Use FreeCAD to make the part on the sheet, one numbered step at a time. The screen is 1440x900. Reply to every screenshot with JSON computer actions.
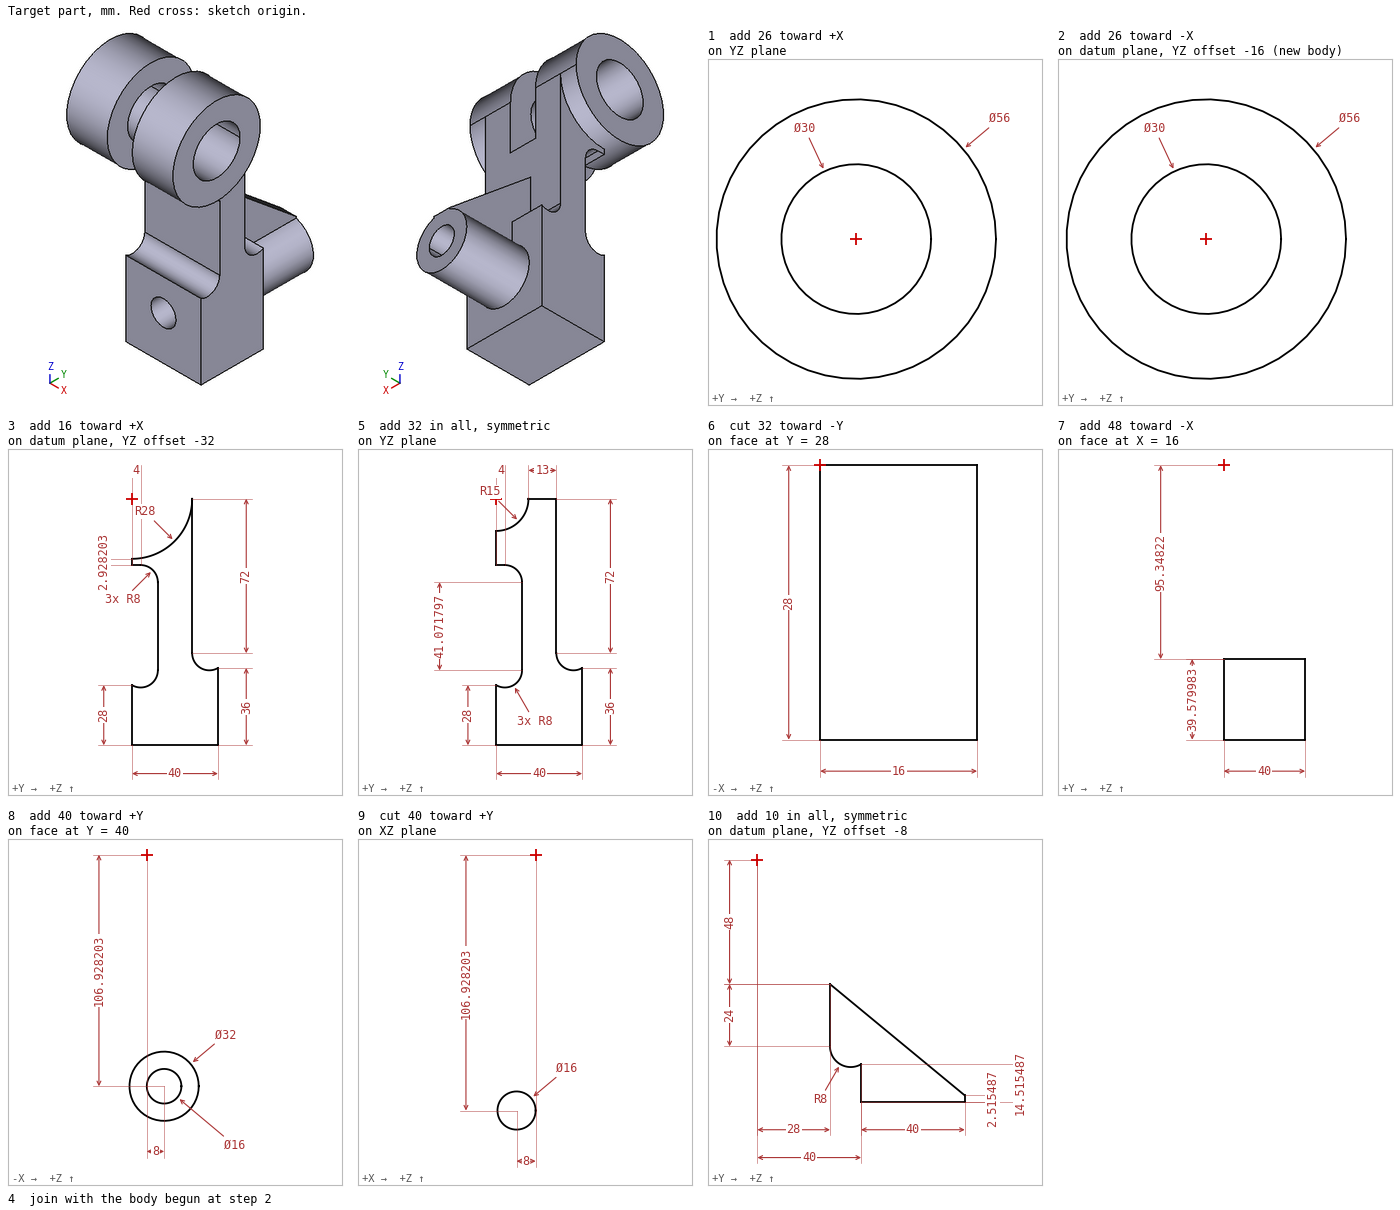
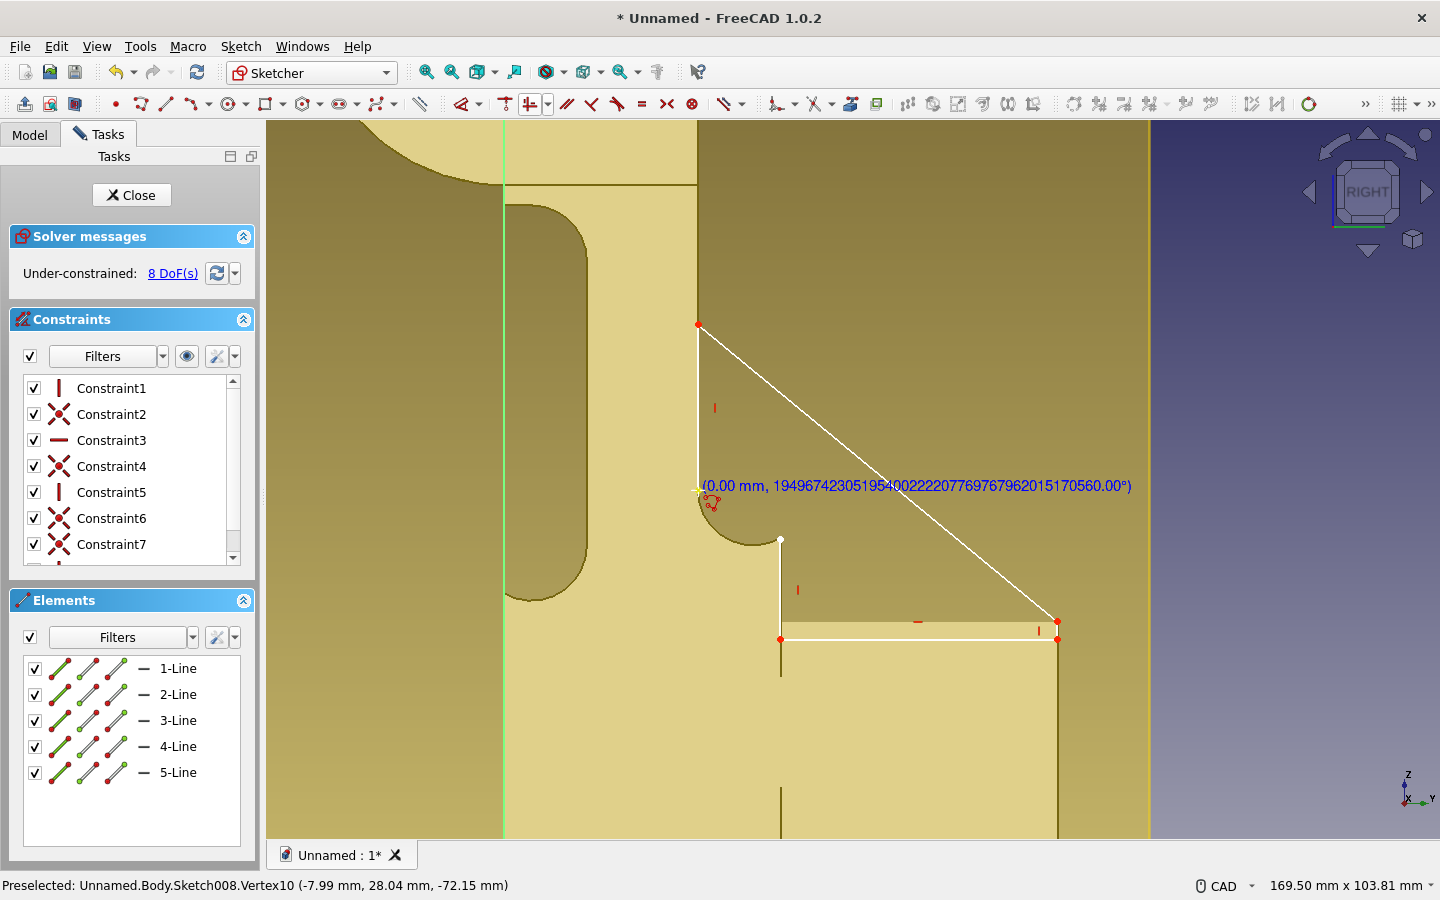
{"action": "key", "text": "g 3 a"}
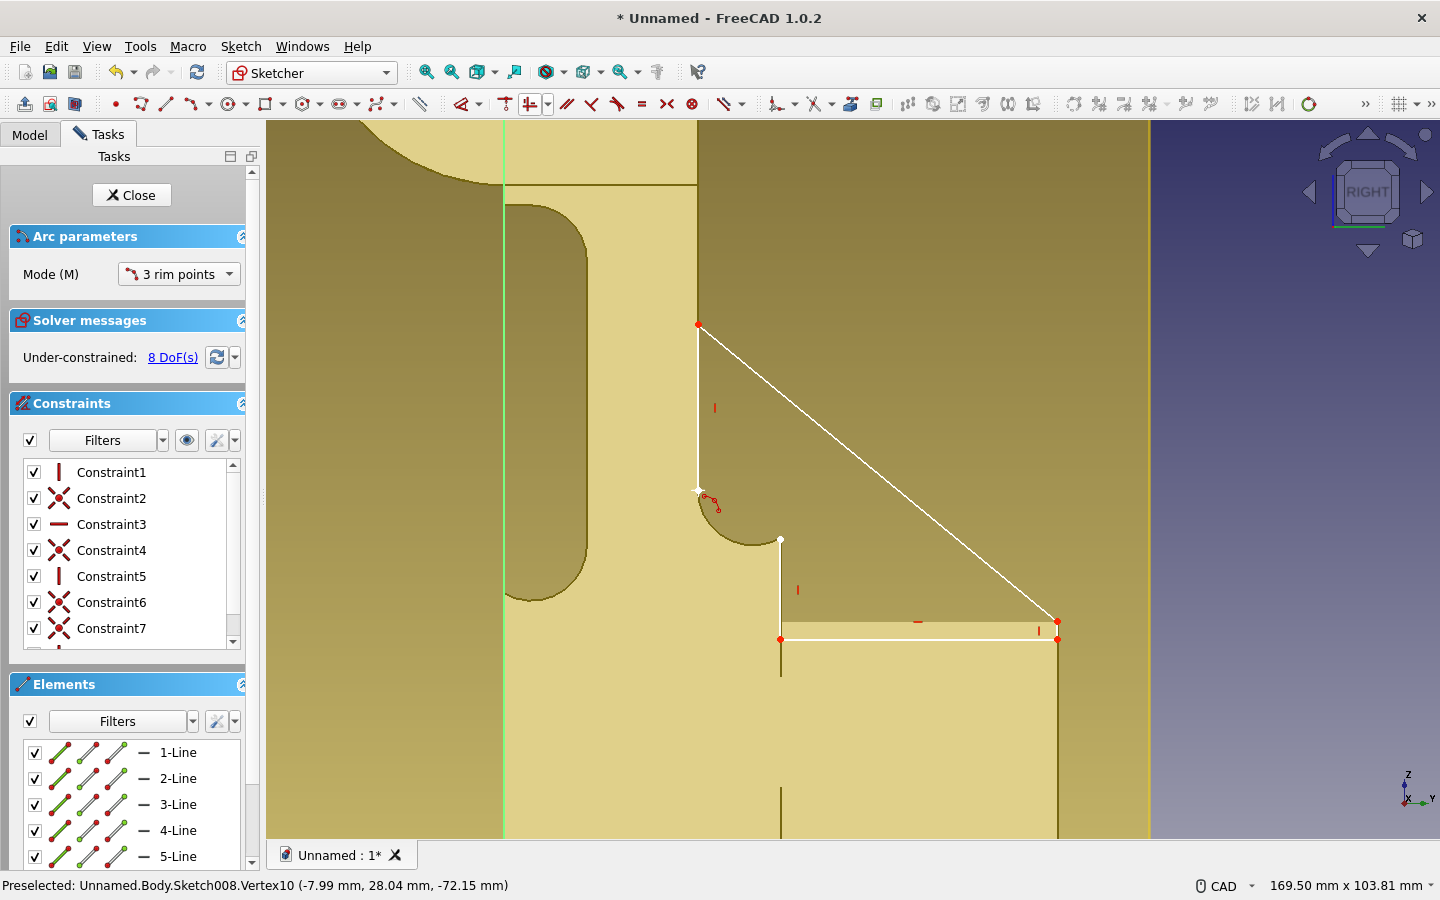
{"action": "left_click", "coordinate": [698, 491]}
{"action": "left_click", "coordinate": [780, 539]}
{"action": "left_click", "coordinate": [725, 538]}
{"action": "key", "text": "Escape"}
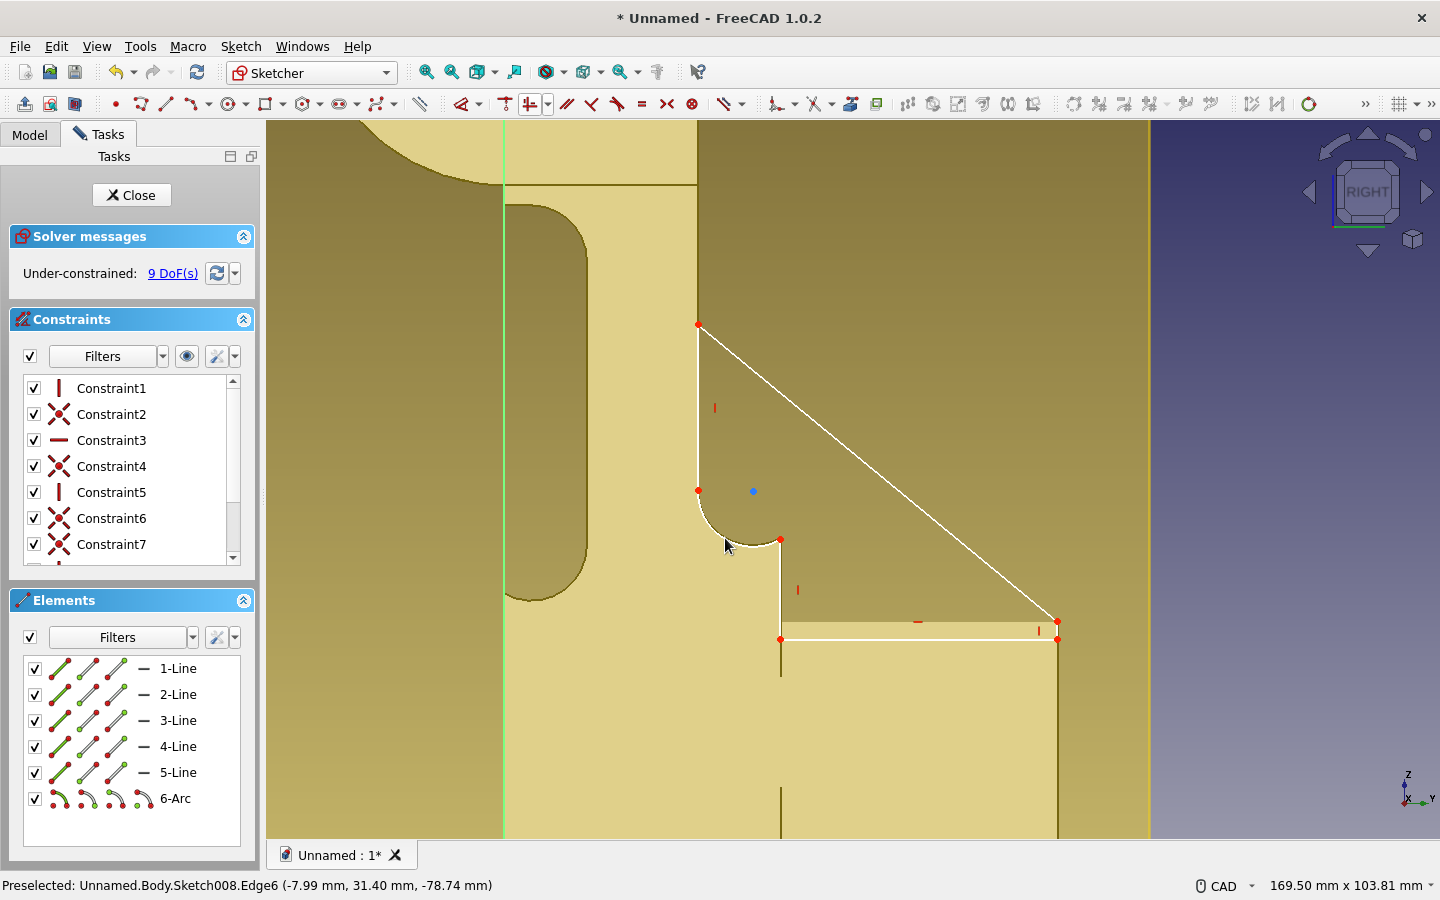
{"action": "left_click", "coordinate": [698, 375]}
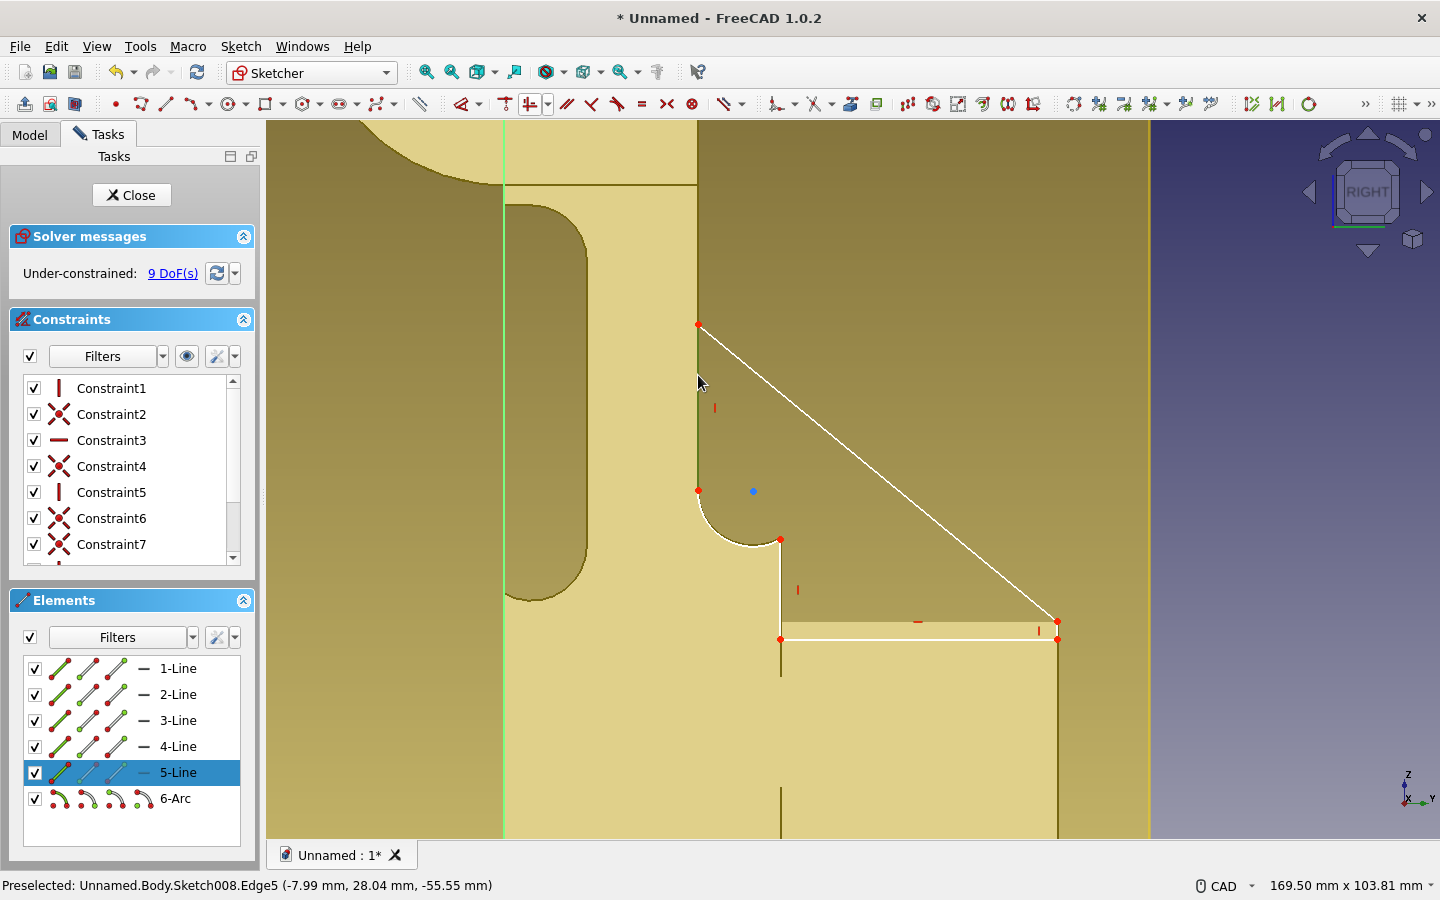
{"action": "left_click", "coordinate": [708, 524]}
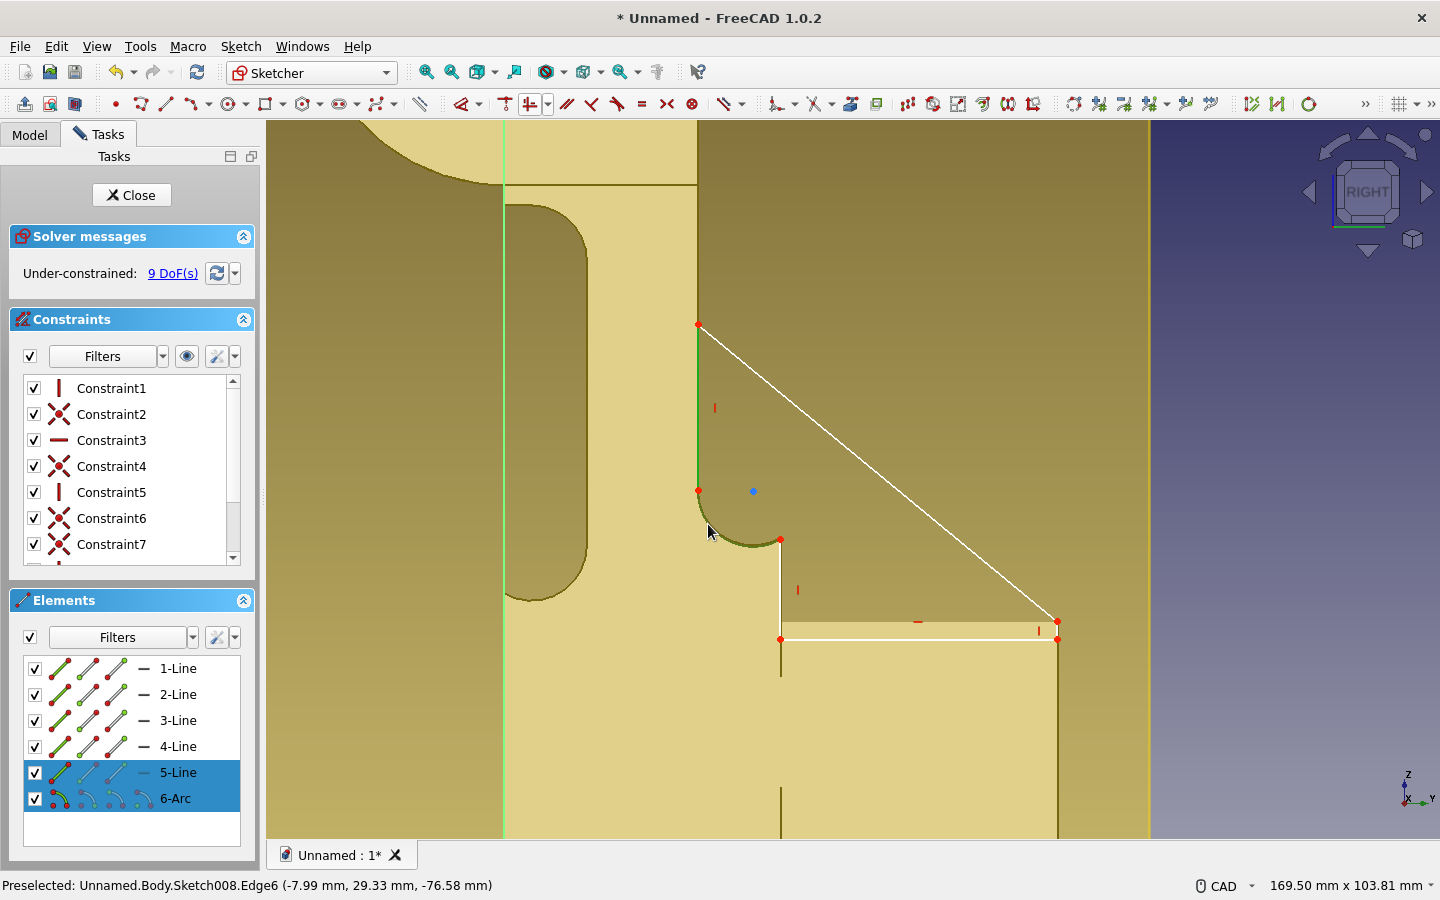
{"action": "left_click", "coordinate": [617, 104]}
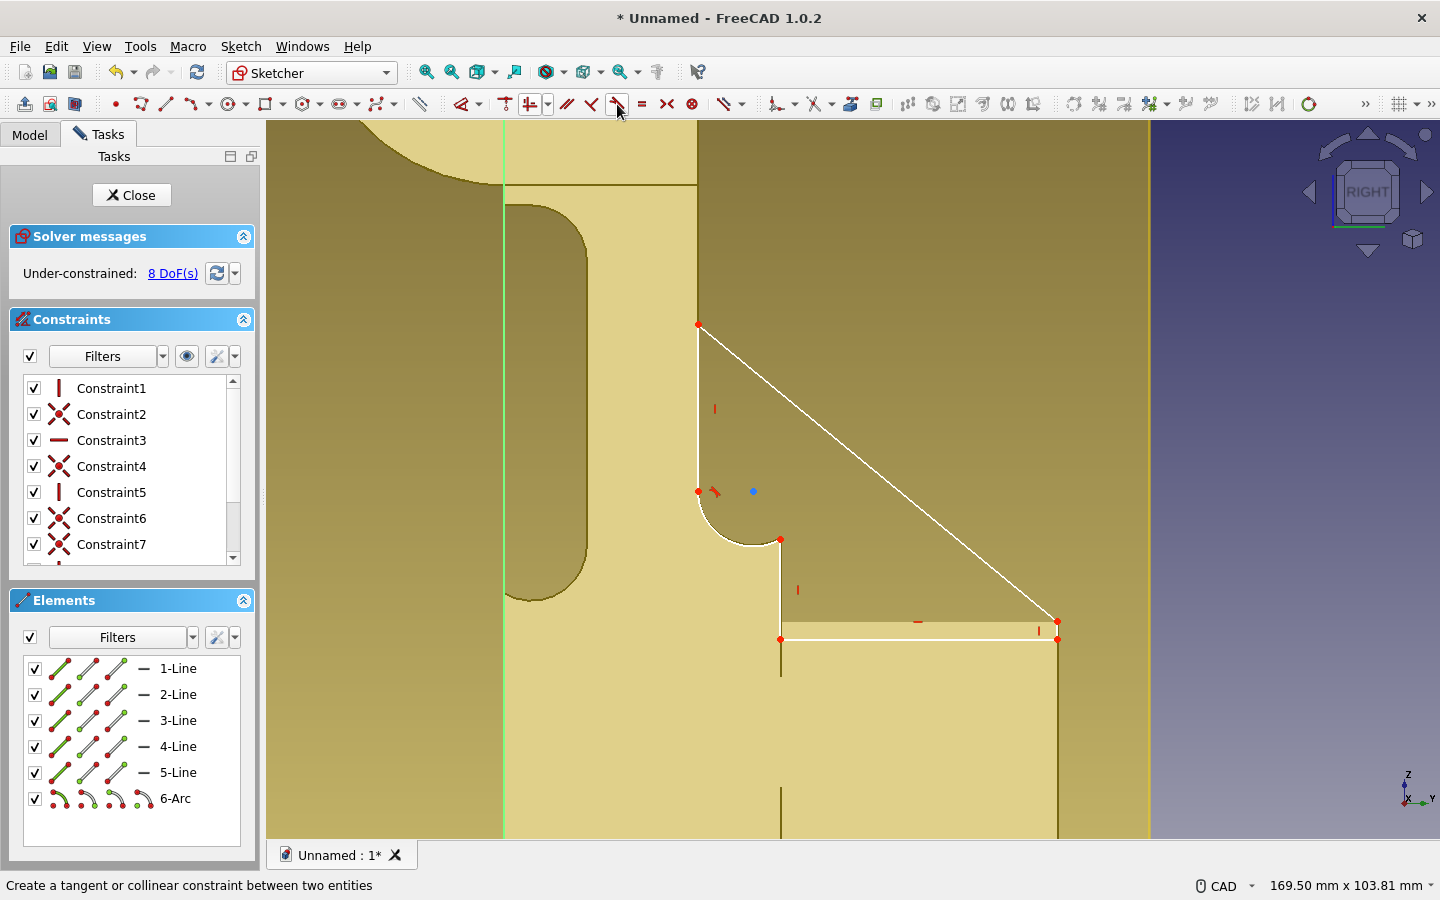
{"action": "key", "text": "d"}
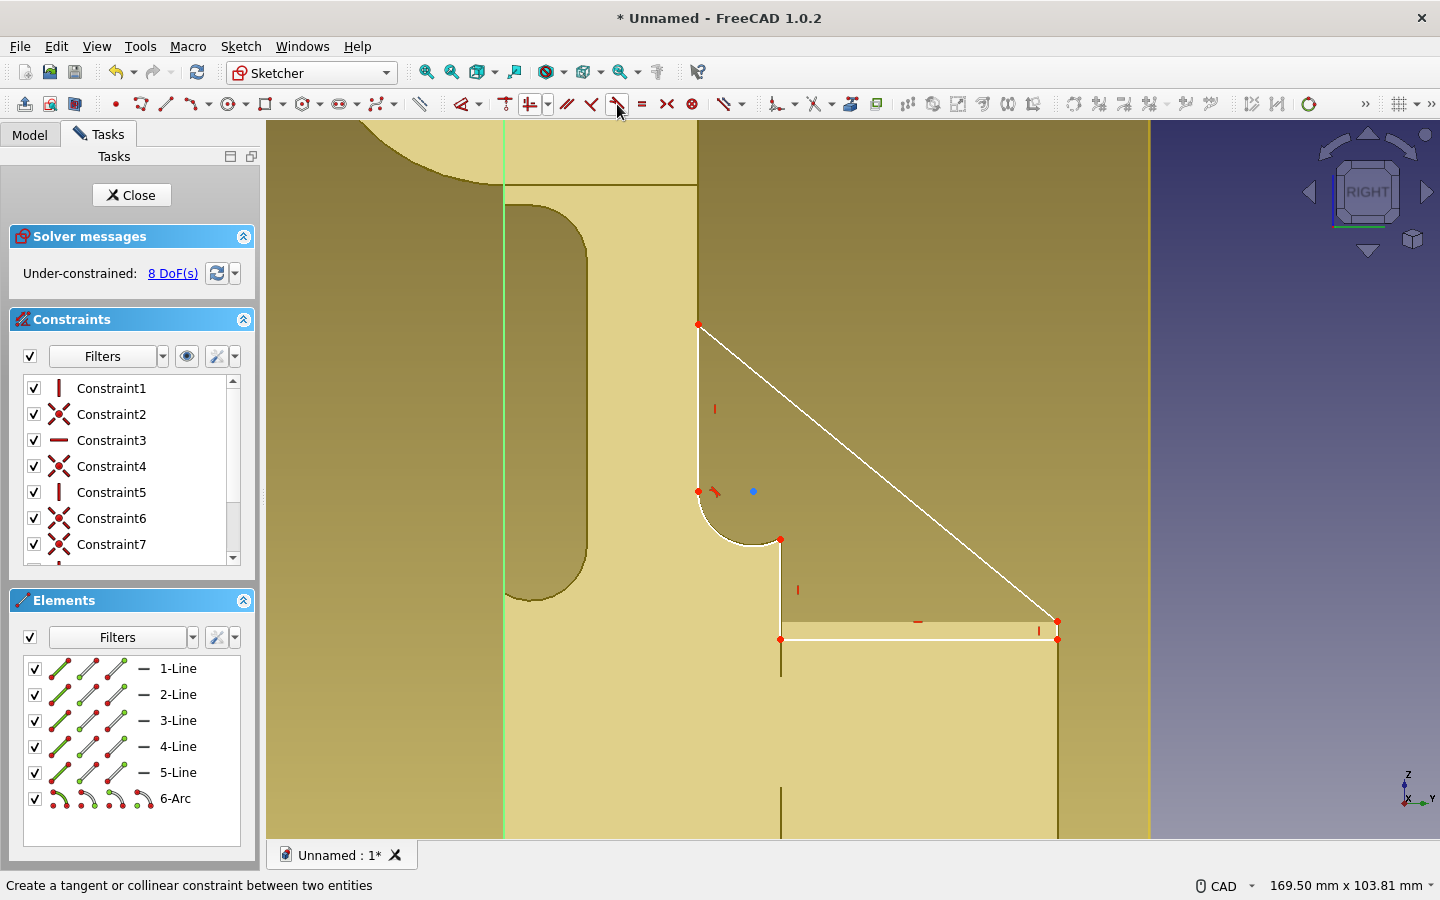
{"action": "left_click", "coordinate": [708, 523]}
{"action": "left_click", "coordinate": [682, 541]}